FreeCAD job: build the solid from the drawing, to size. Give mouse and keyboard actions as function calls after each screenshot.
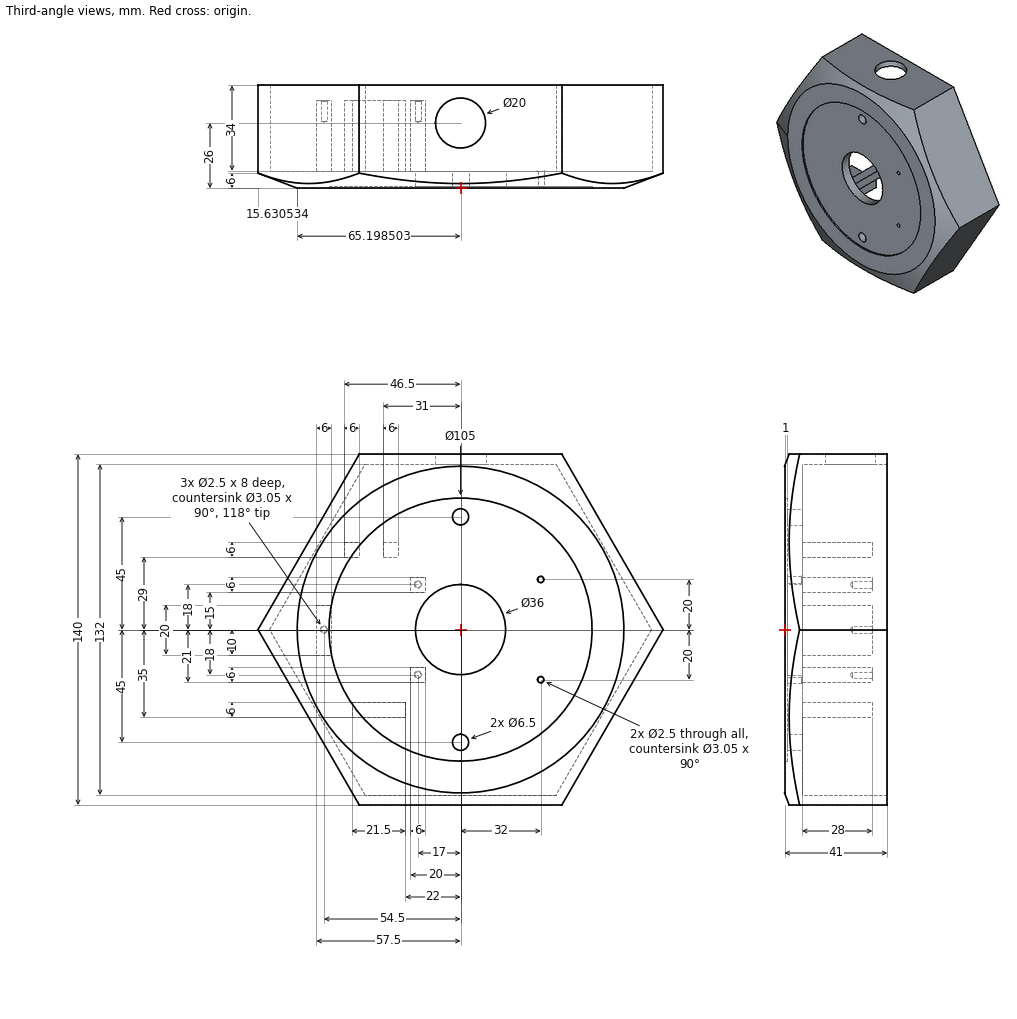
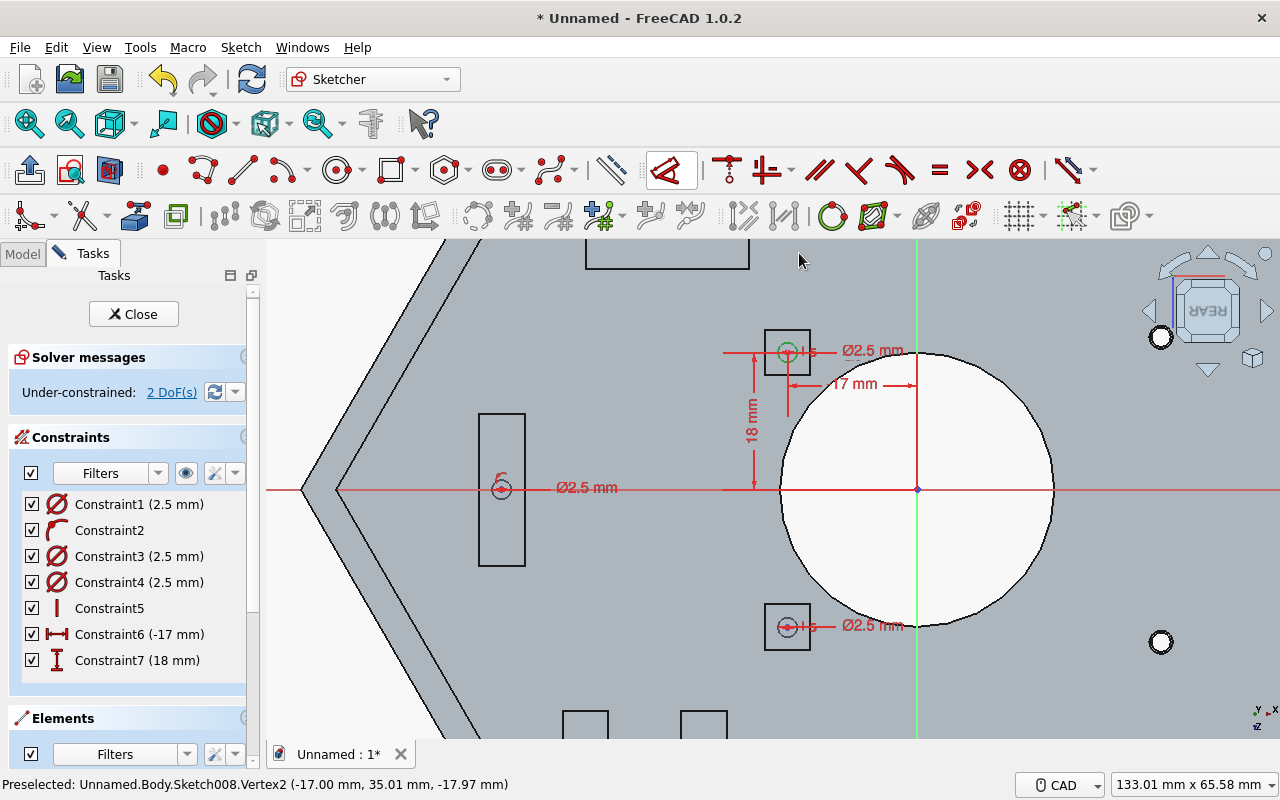
click(788, 627)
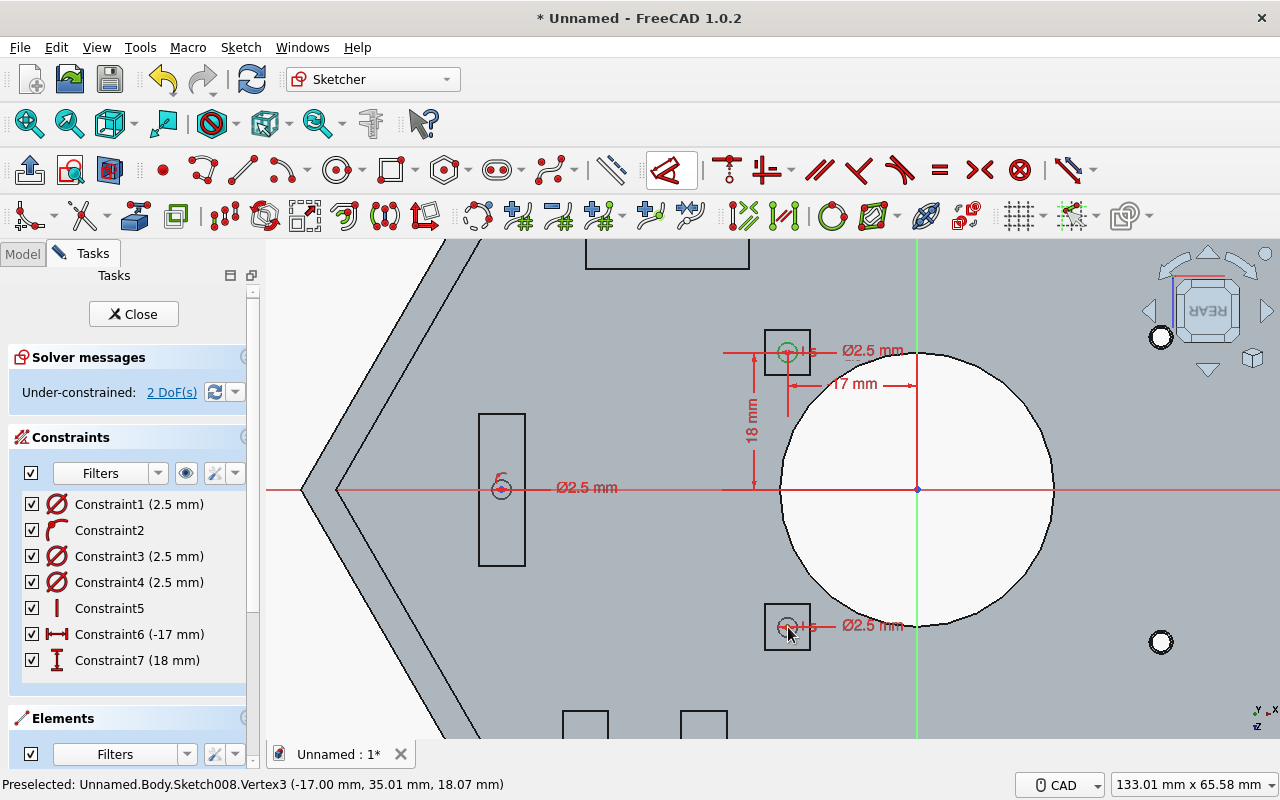
click(692, 170)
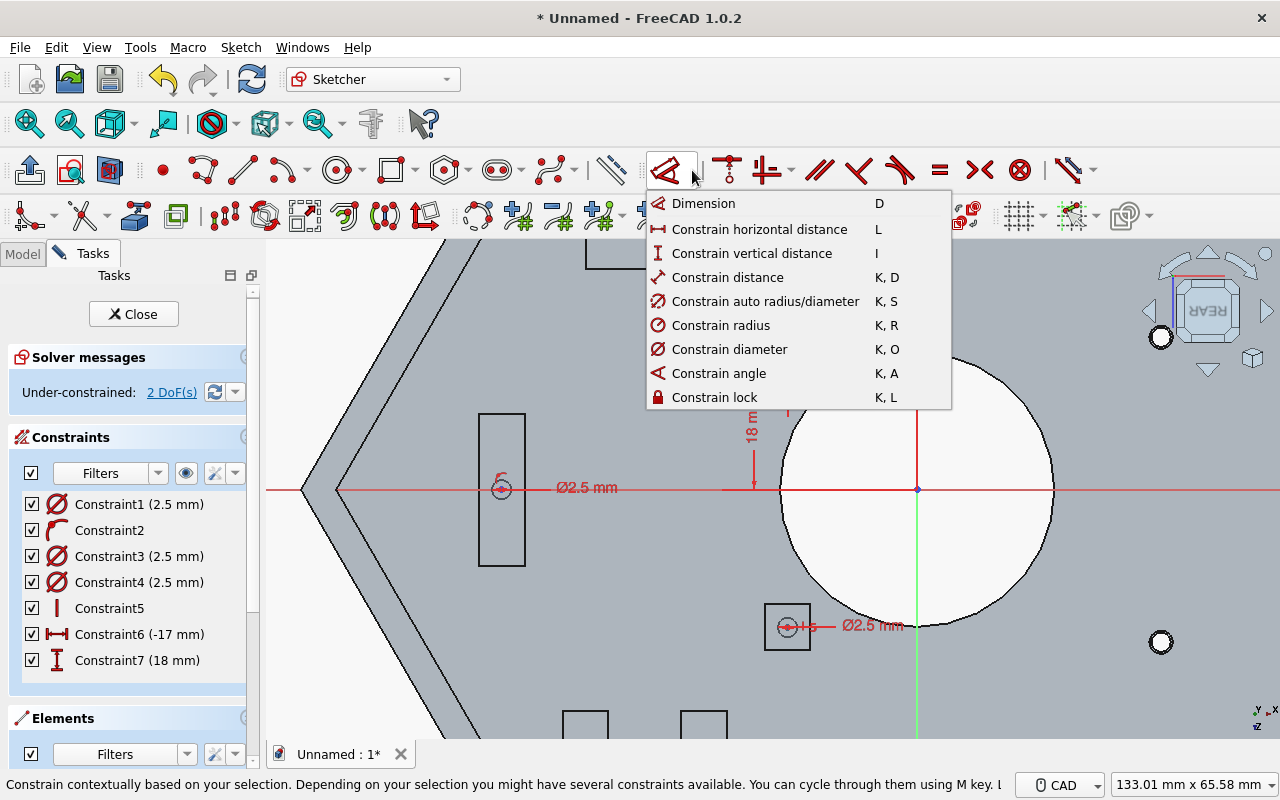
click(799, 253)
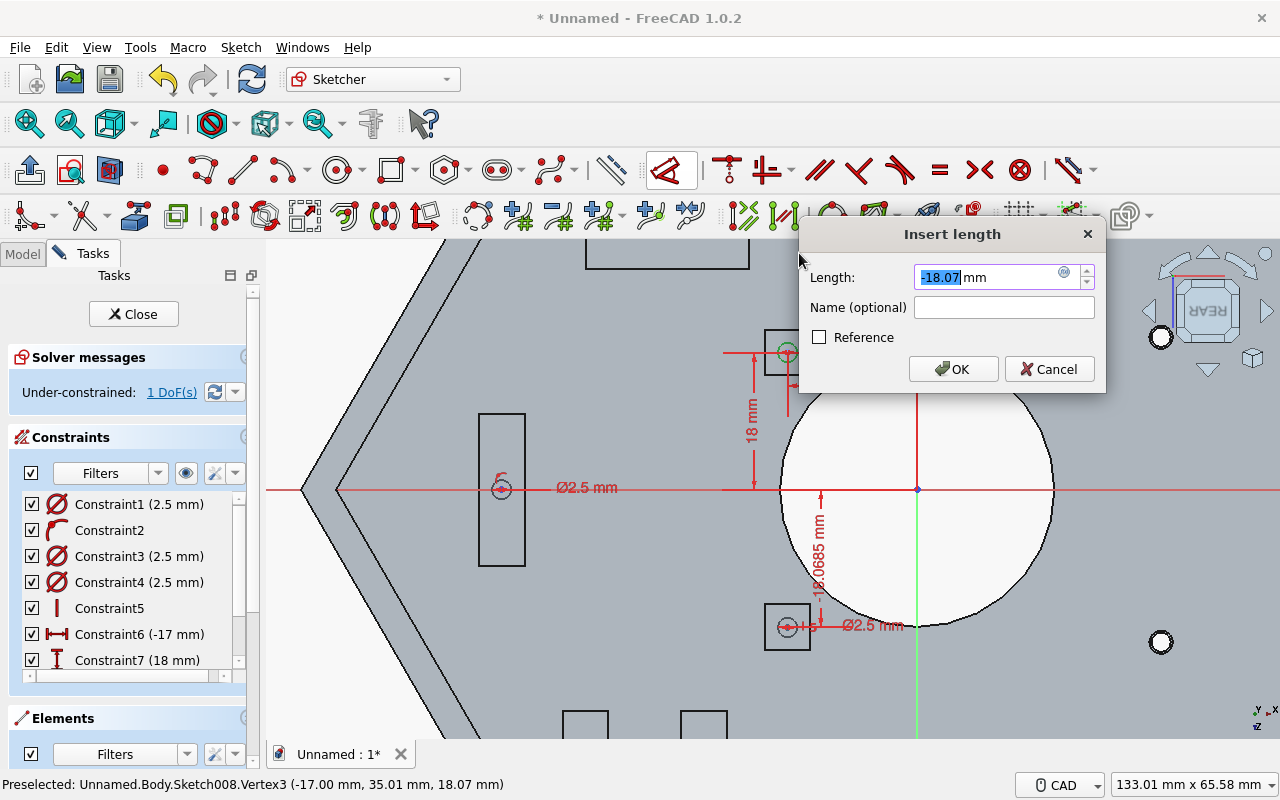
text(-18)
key(Return)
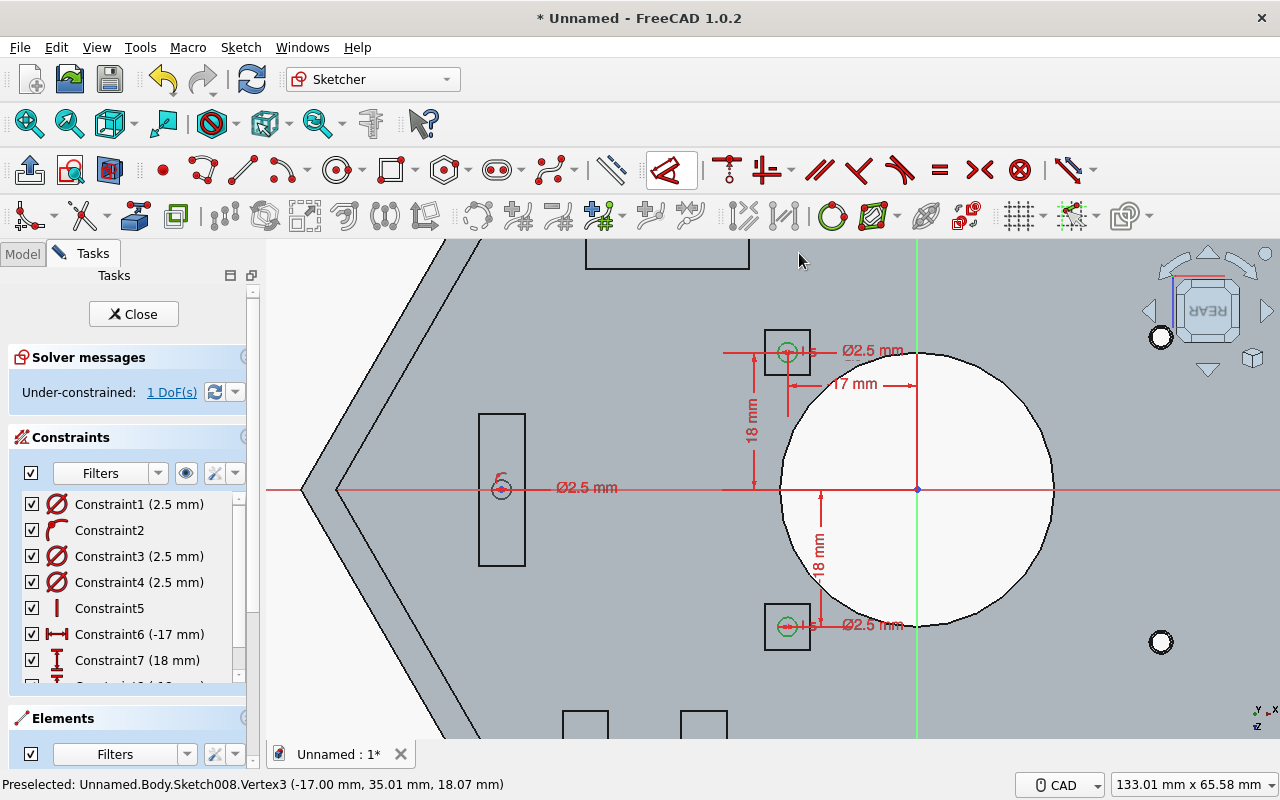
click(502, 490)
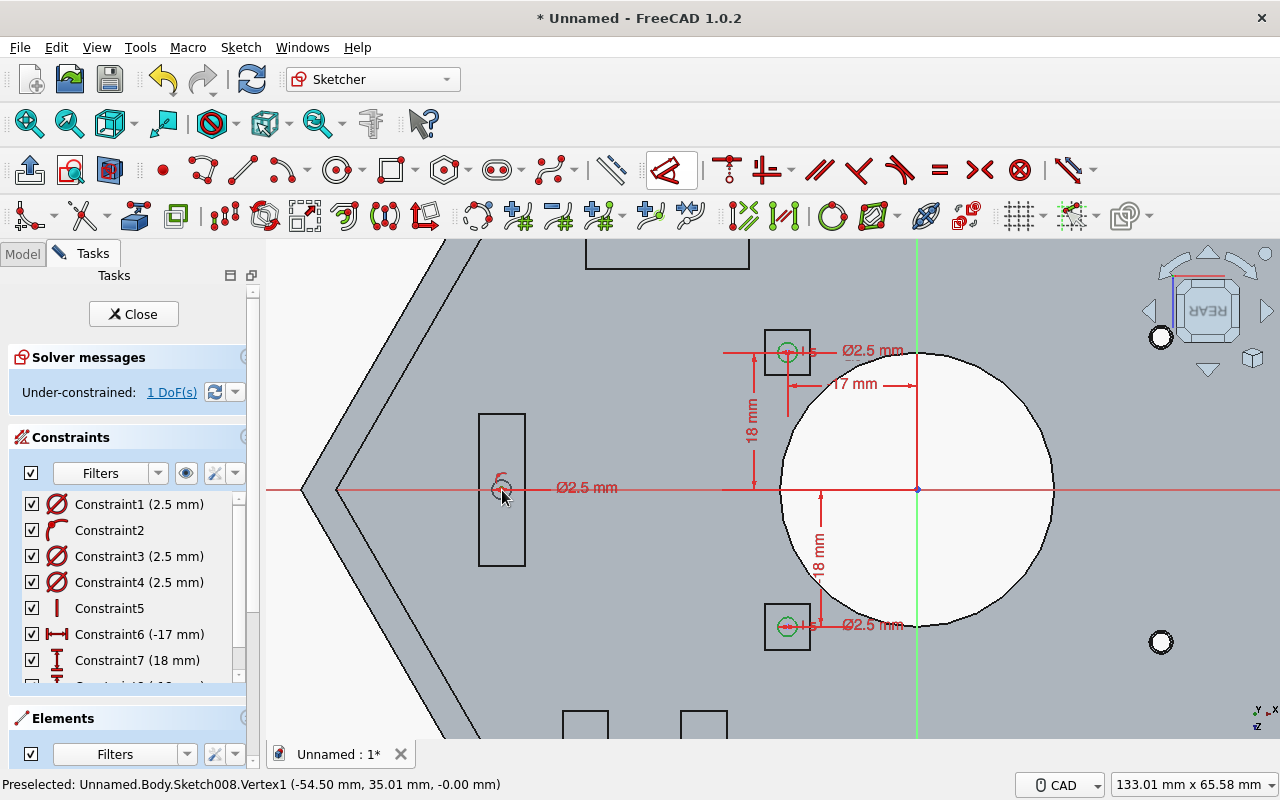
key(l)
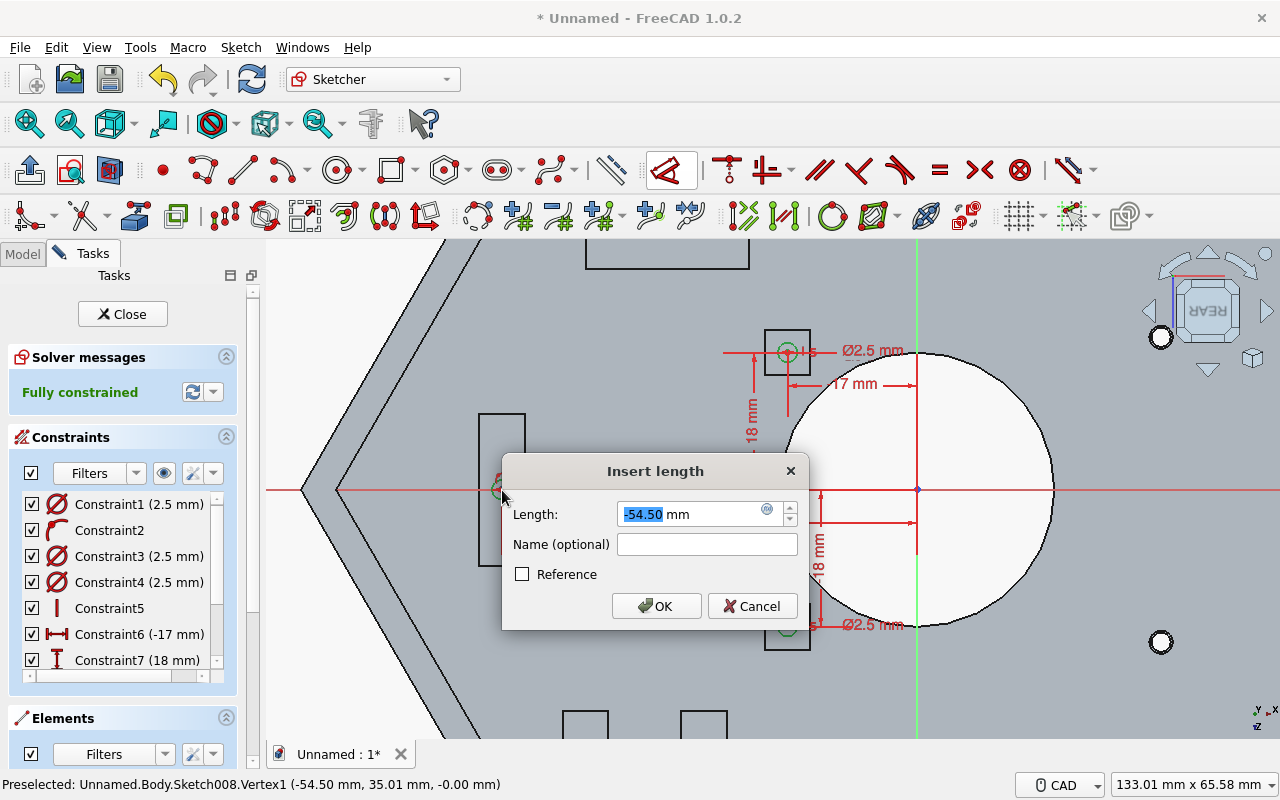
text(-54.5)
key(Return)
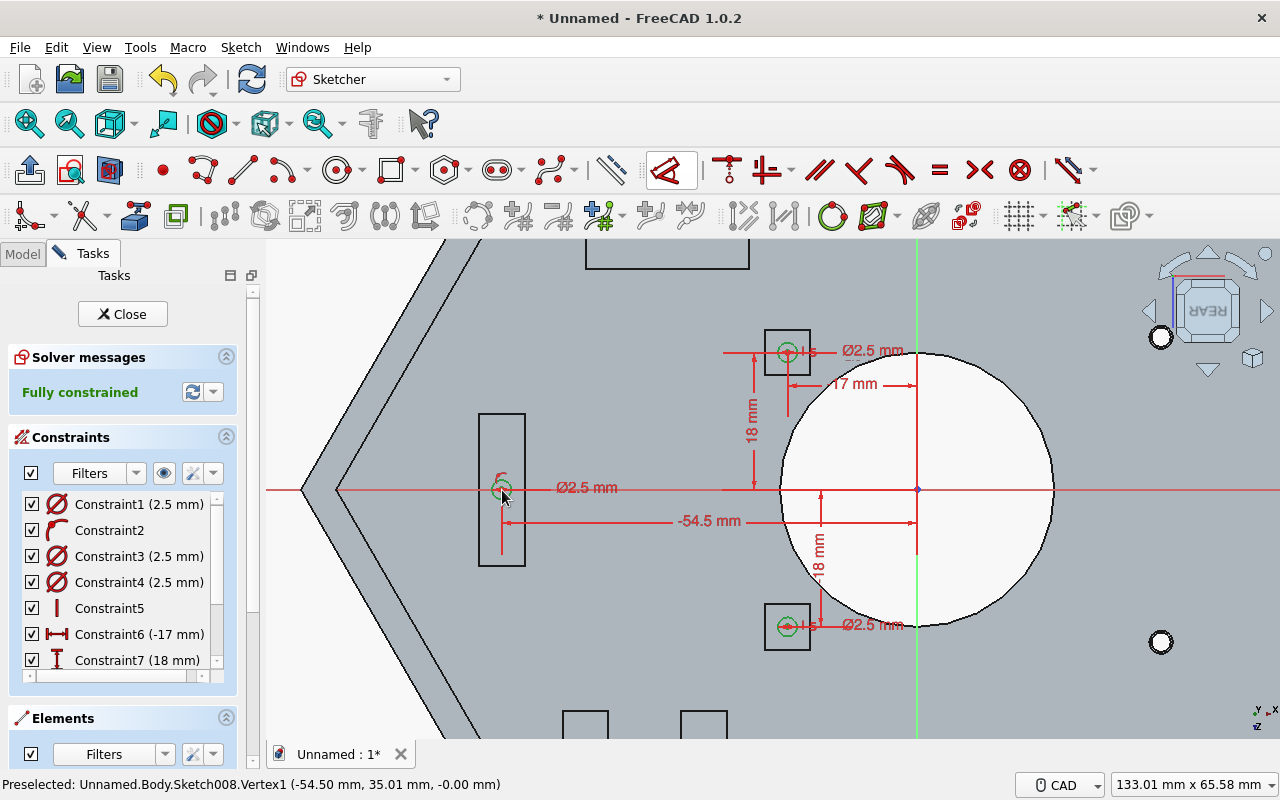
click(123, 314)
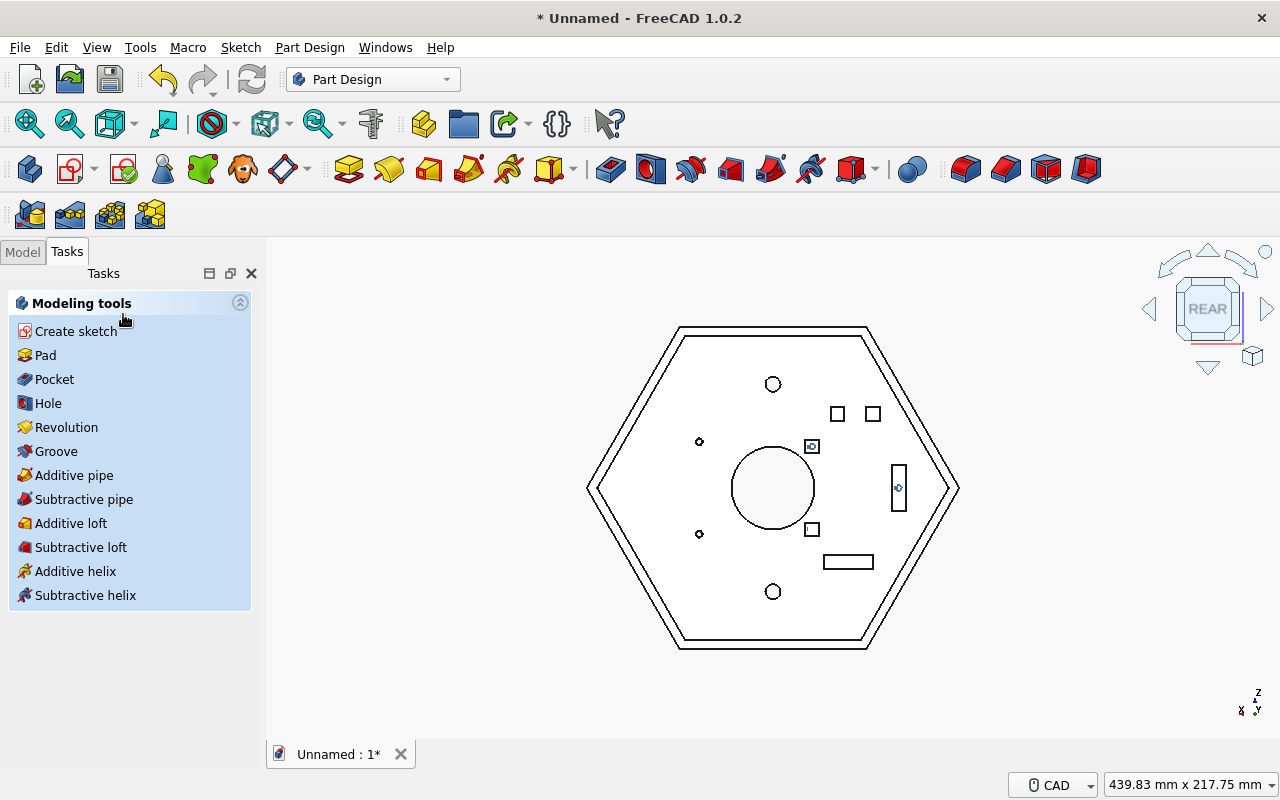
click(652, 170)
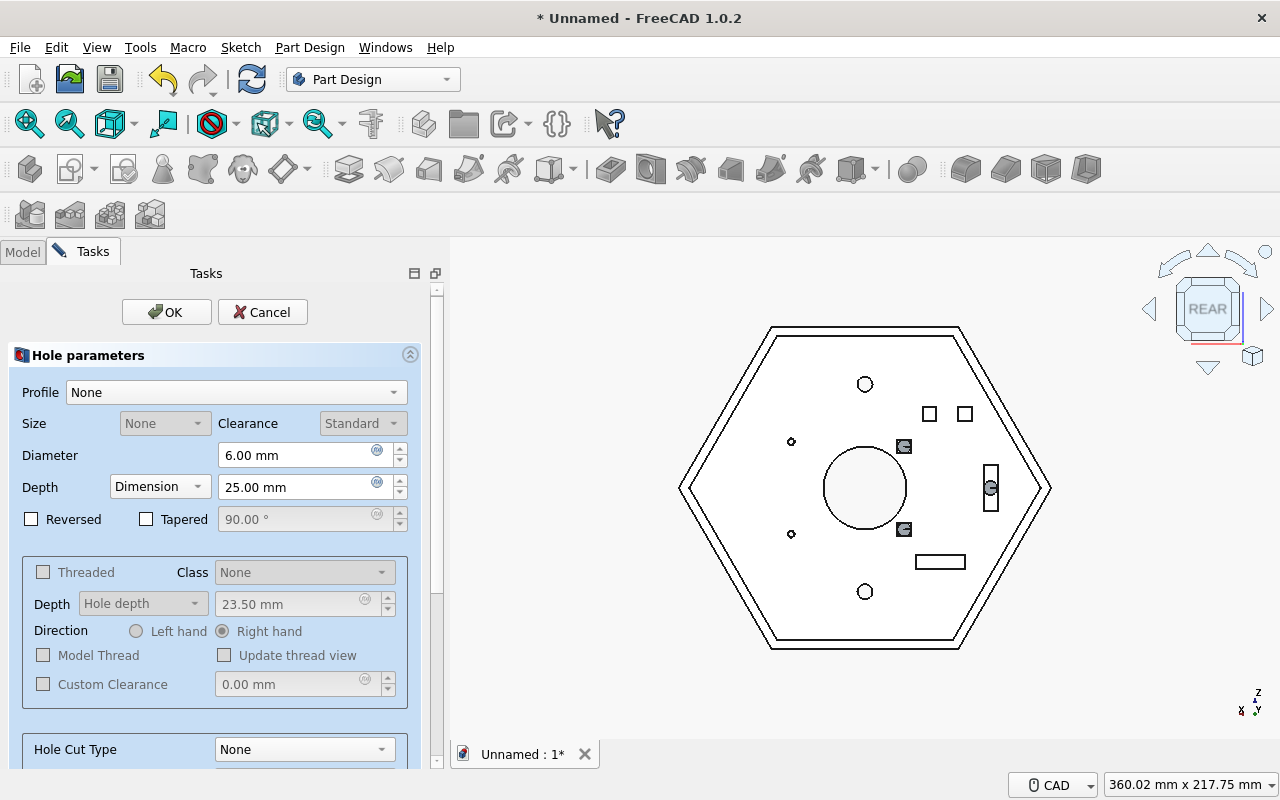
triple_click(305, 455)